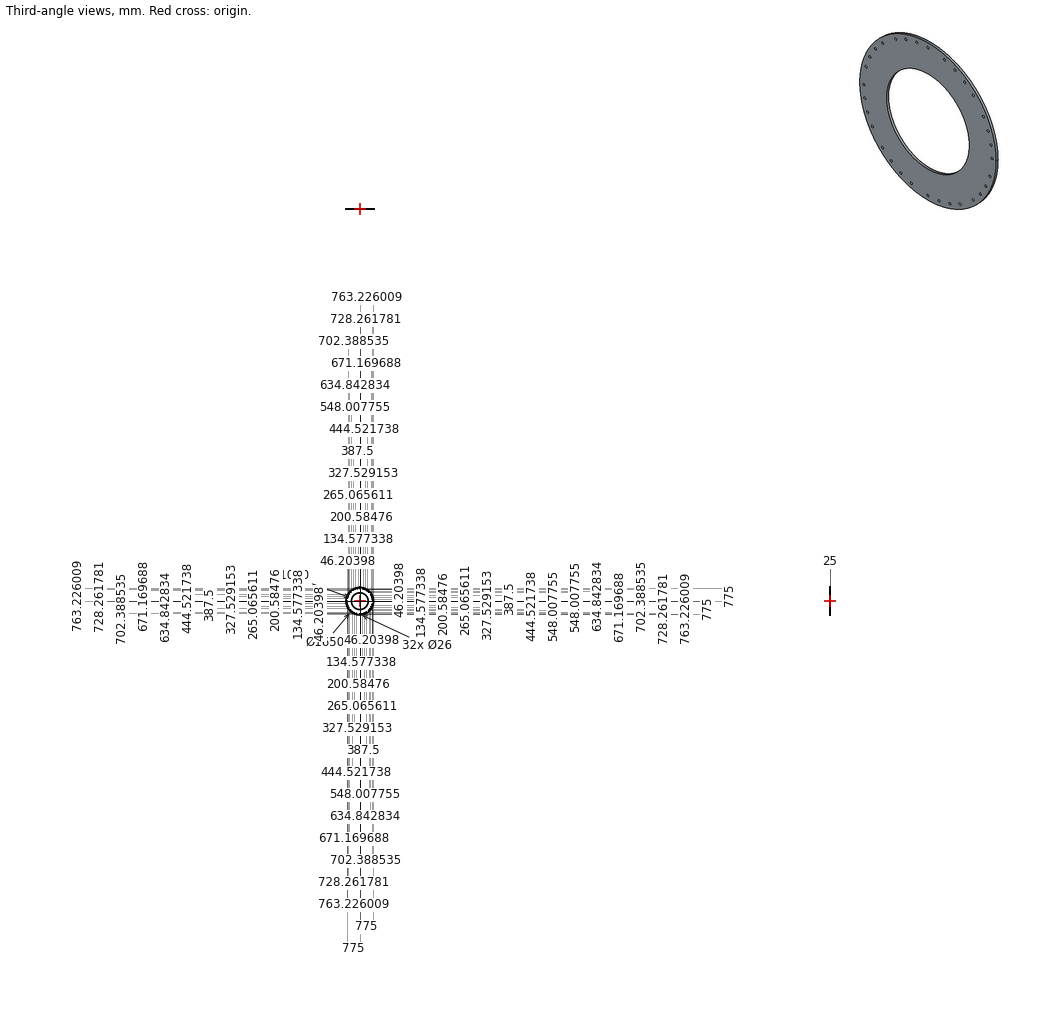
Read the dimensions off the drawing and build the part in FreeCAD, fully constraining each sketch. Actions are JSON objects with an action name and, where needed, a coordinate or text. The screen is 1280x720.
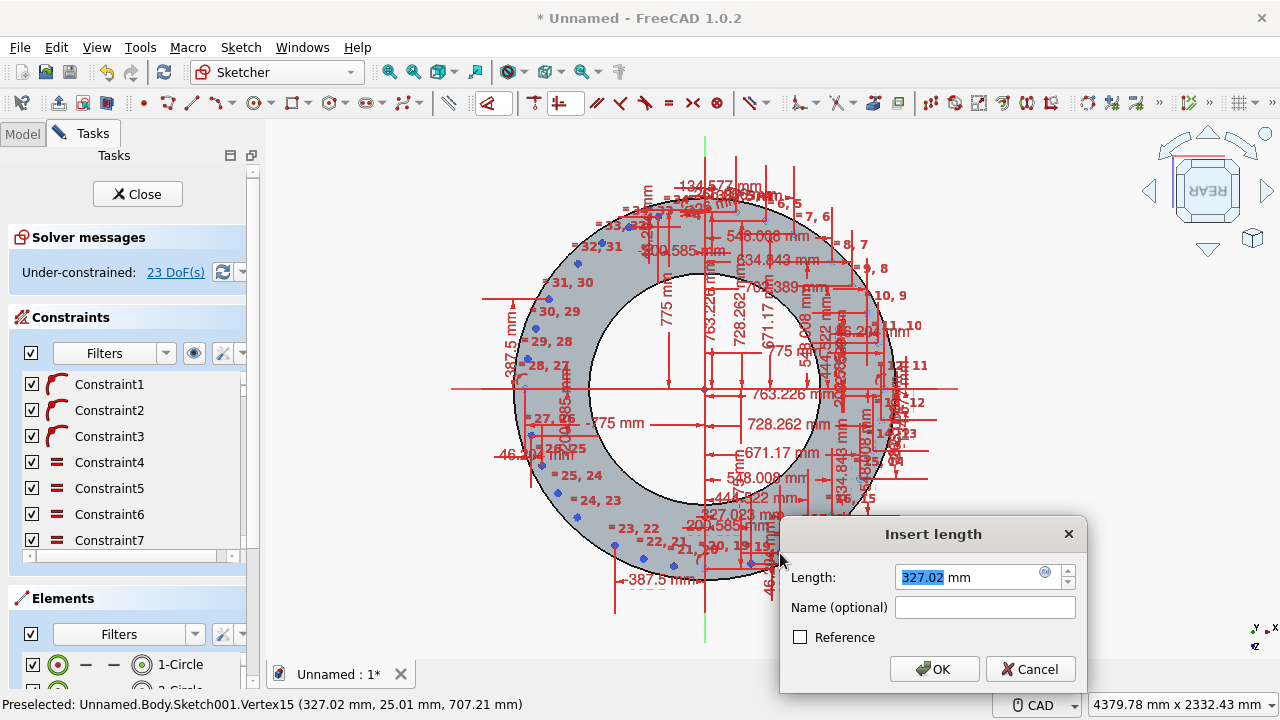
{"action": "type", "text": "327.529153"}
{"action": "key", "text": "Return"}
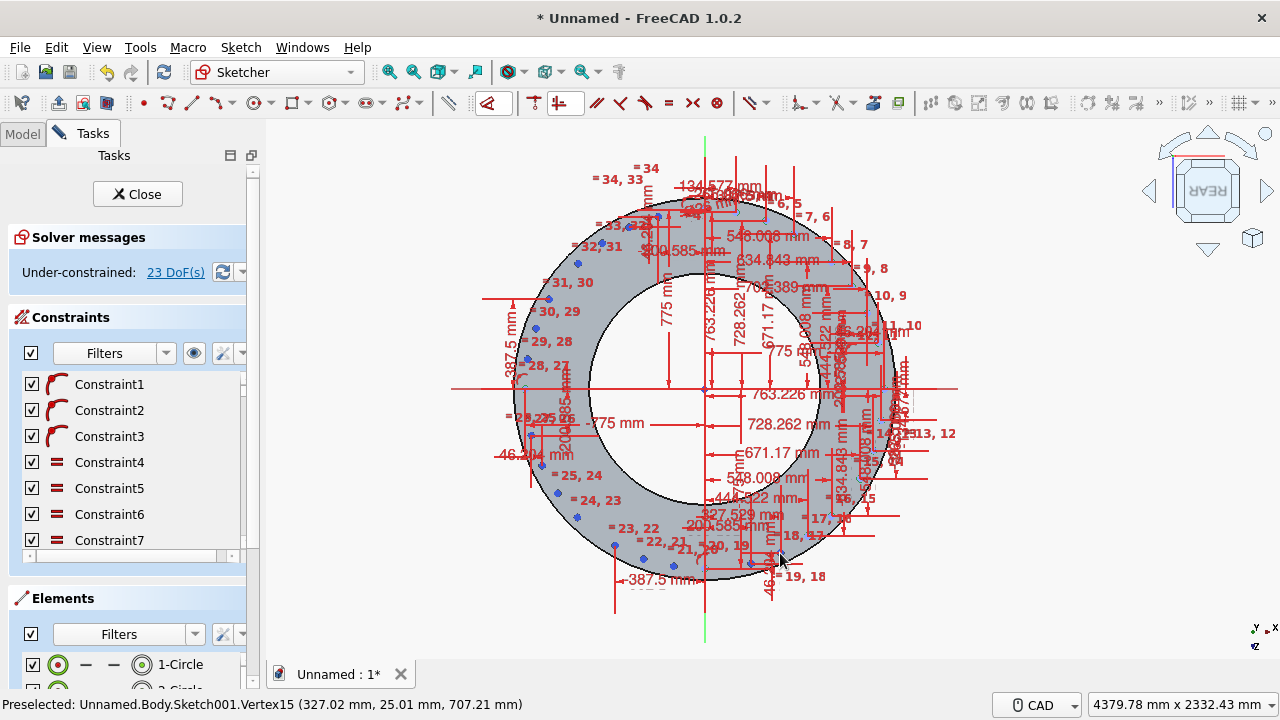
{"action": "left_click", "coordinate": [781, 553]}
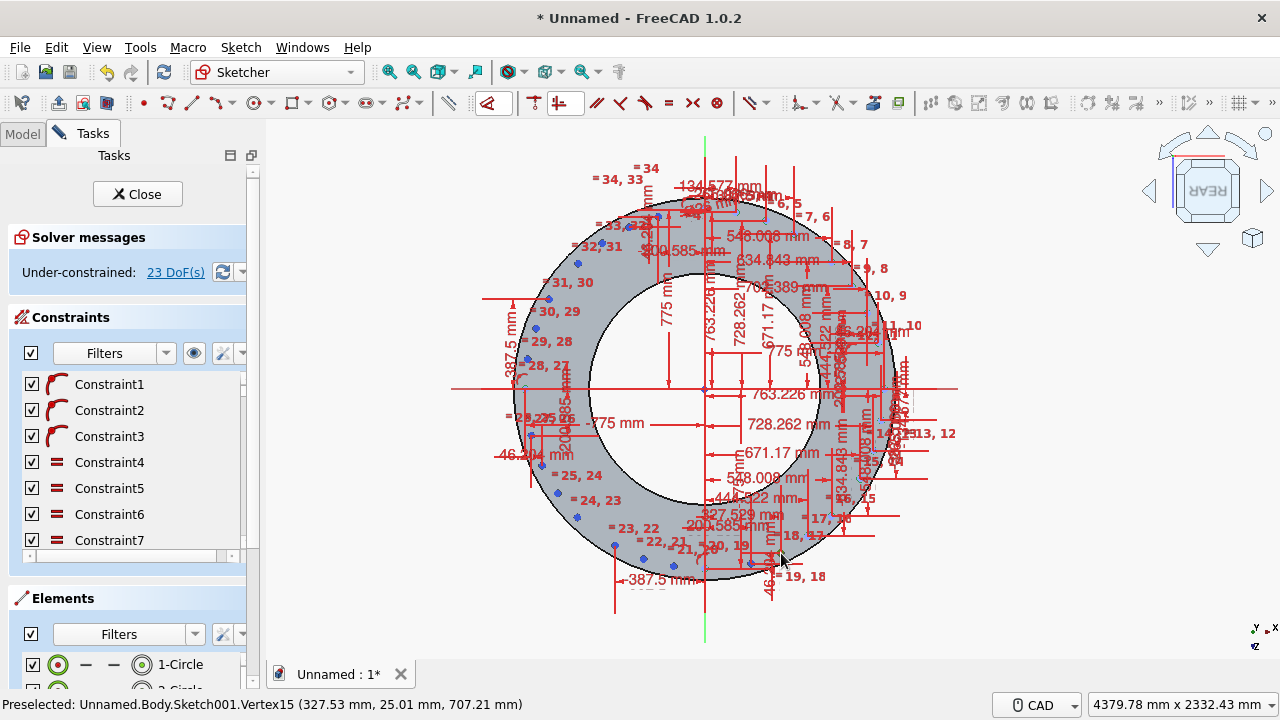
{"action": "key", "text": "i"}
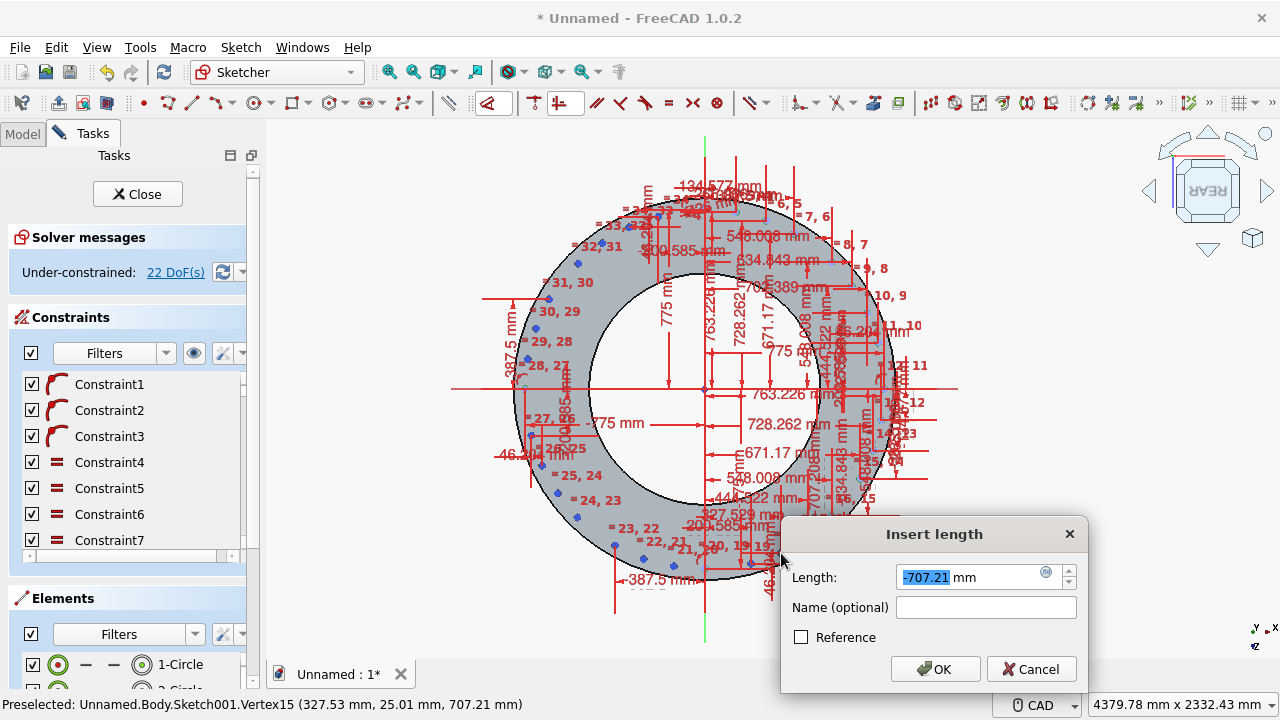
{"action": "type", "text": "-702.388535"}
{"action": "key", "text": "Return"}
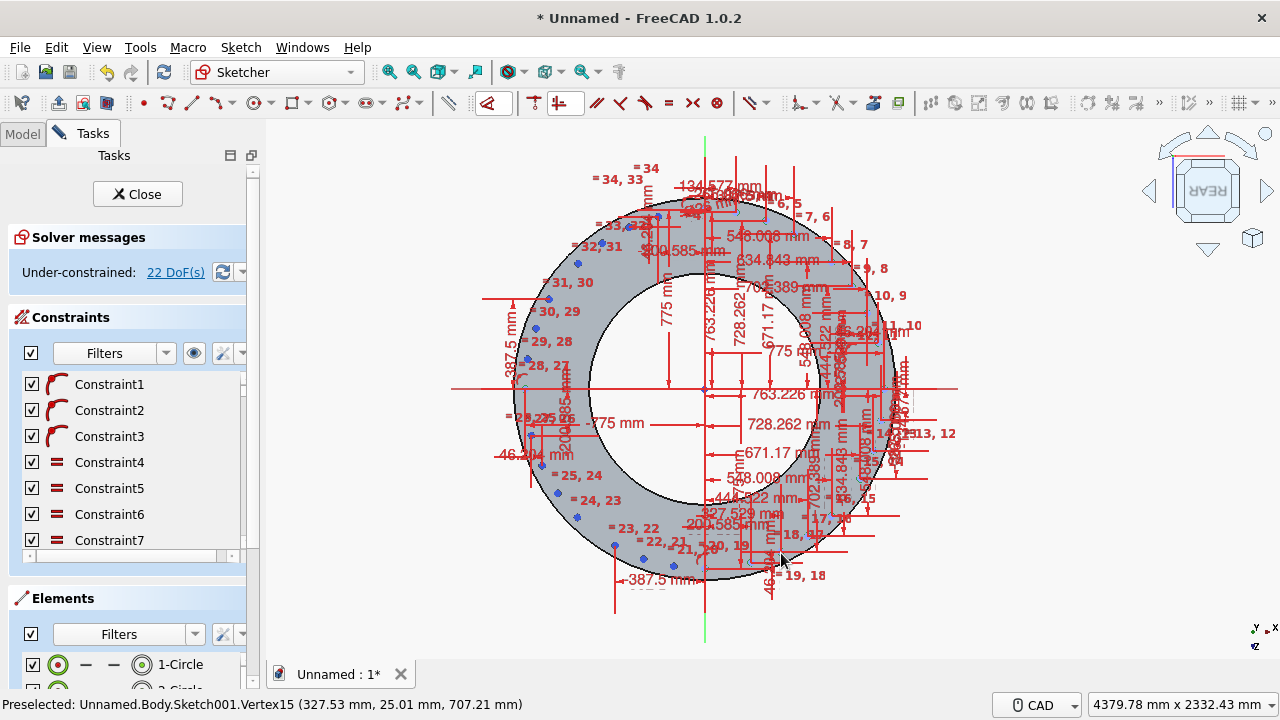
{"action": "scroll", "coordinate": [674, 566], "scroll_direction": "up", "scroll_amount": 2}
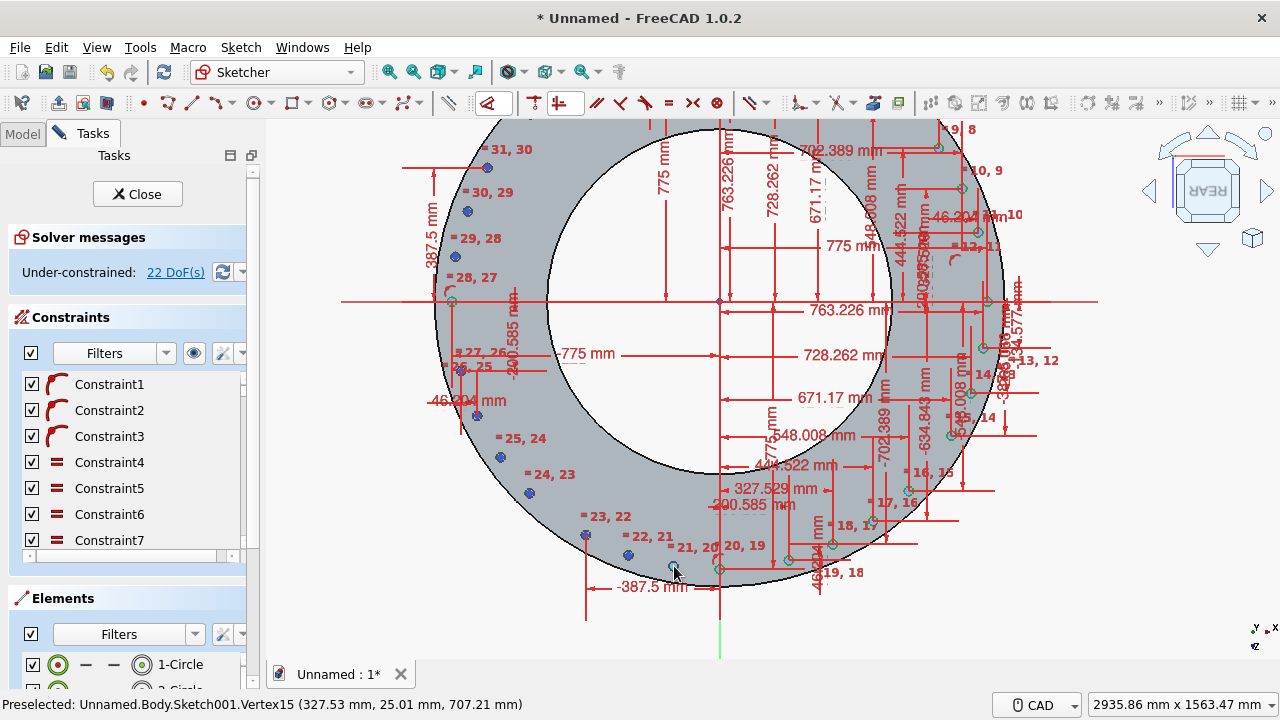
{"action": "left_click", "coordinate": [673, 566]}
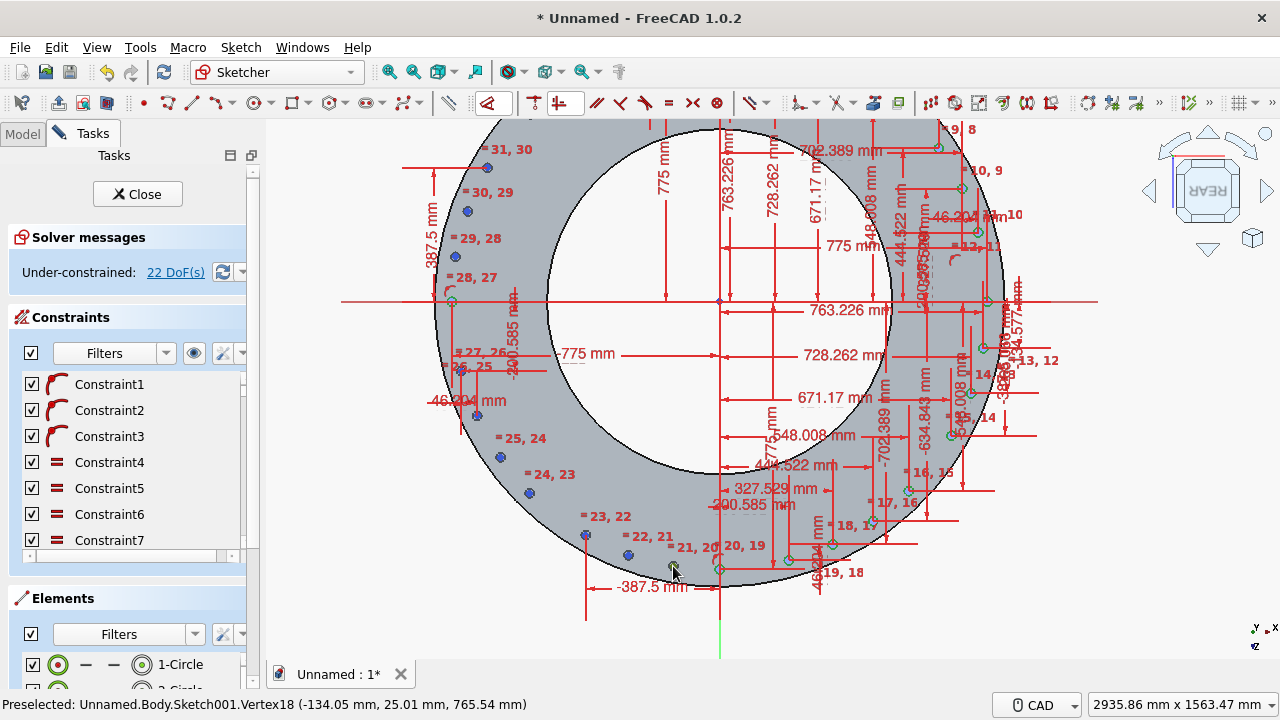
{"action": "key", "text": "l"}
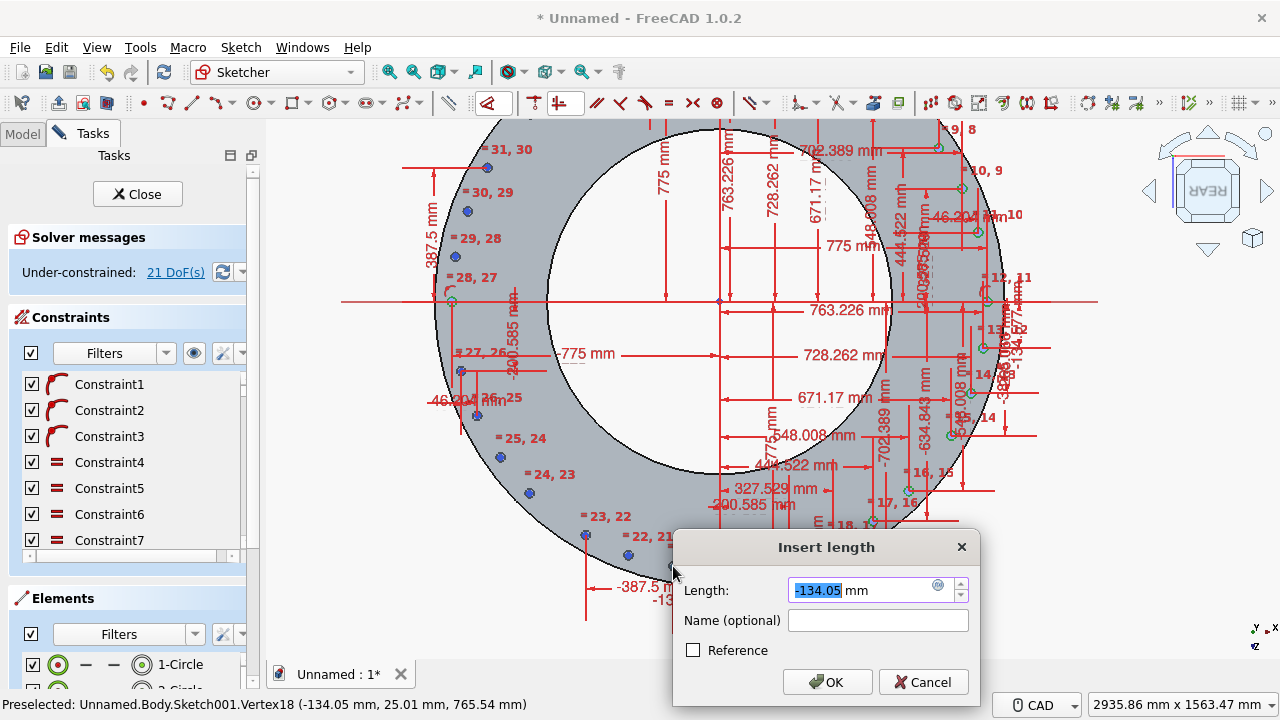
{"action": "type", "text": "-134.577338"}
{"action": "key", "text": "Return"}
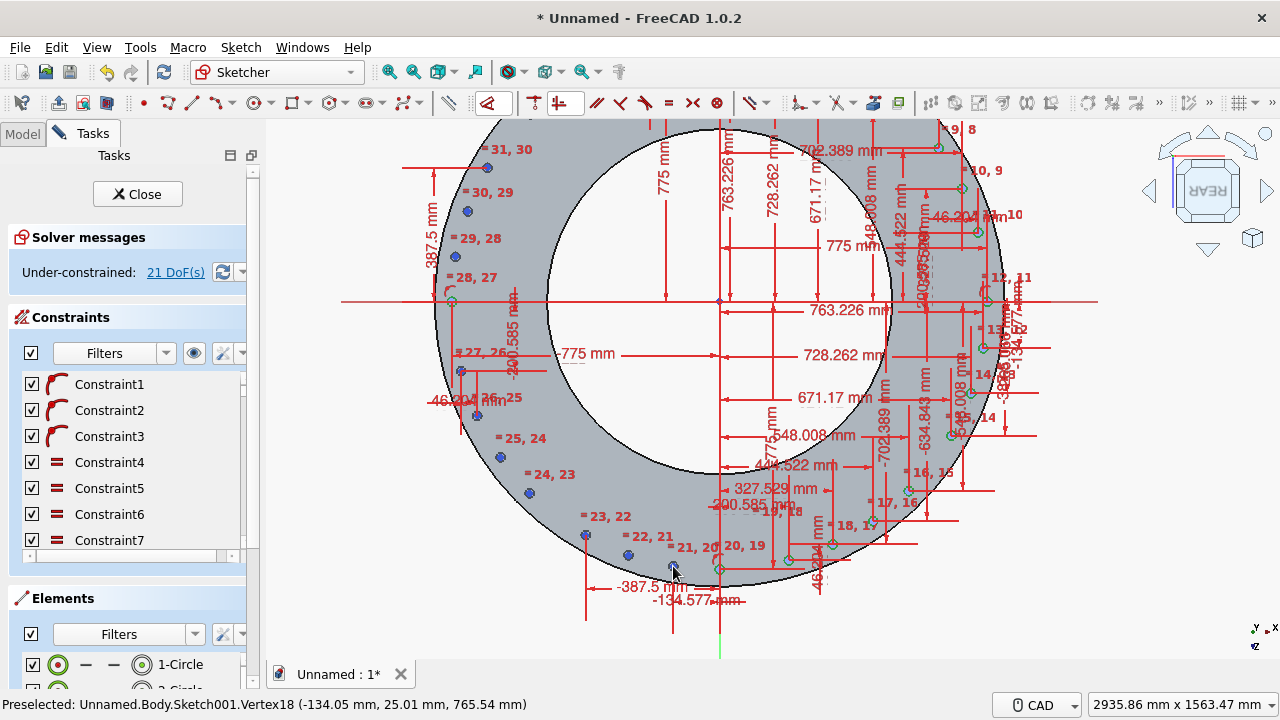
{"action": "left_click", "coordinate": [673, 566]}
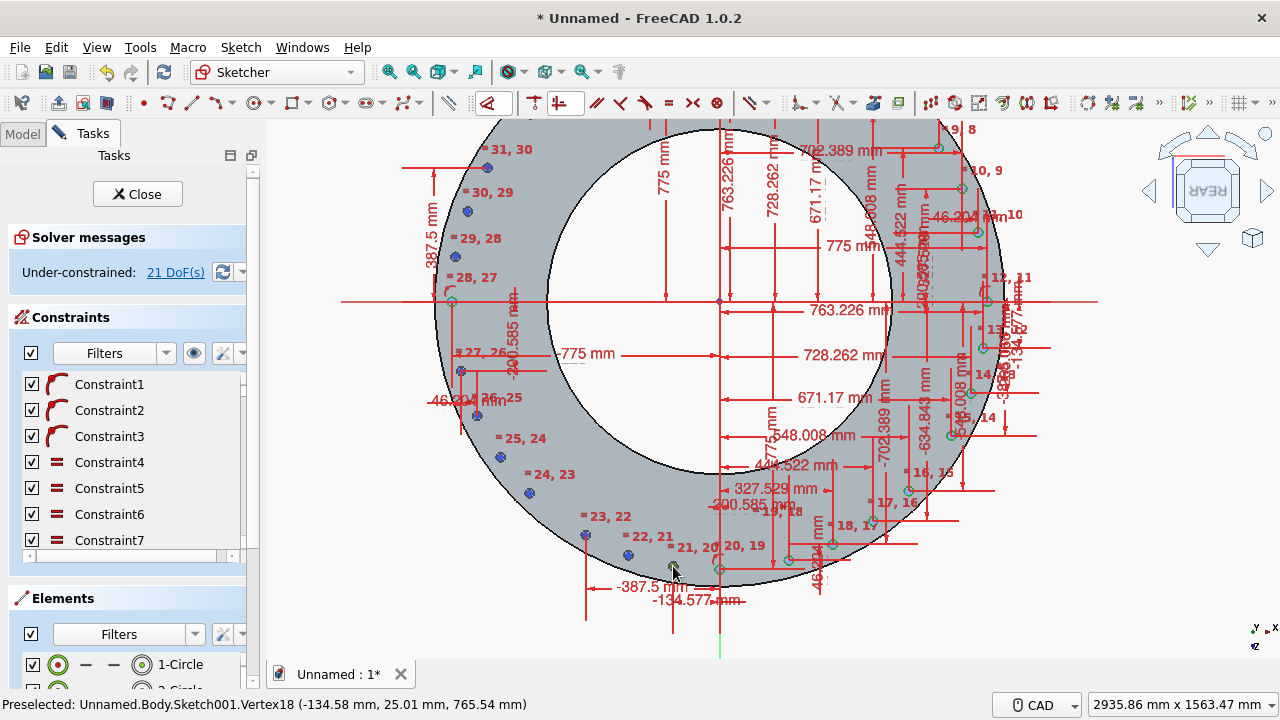
{"action": "key", "text": "i"}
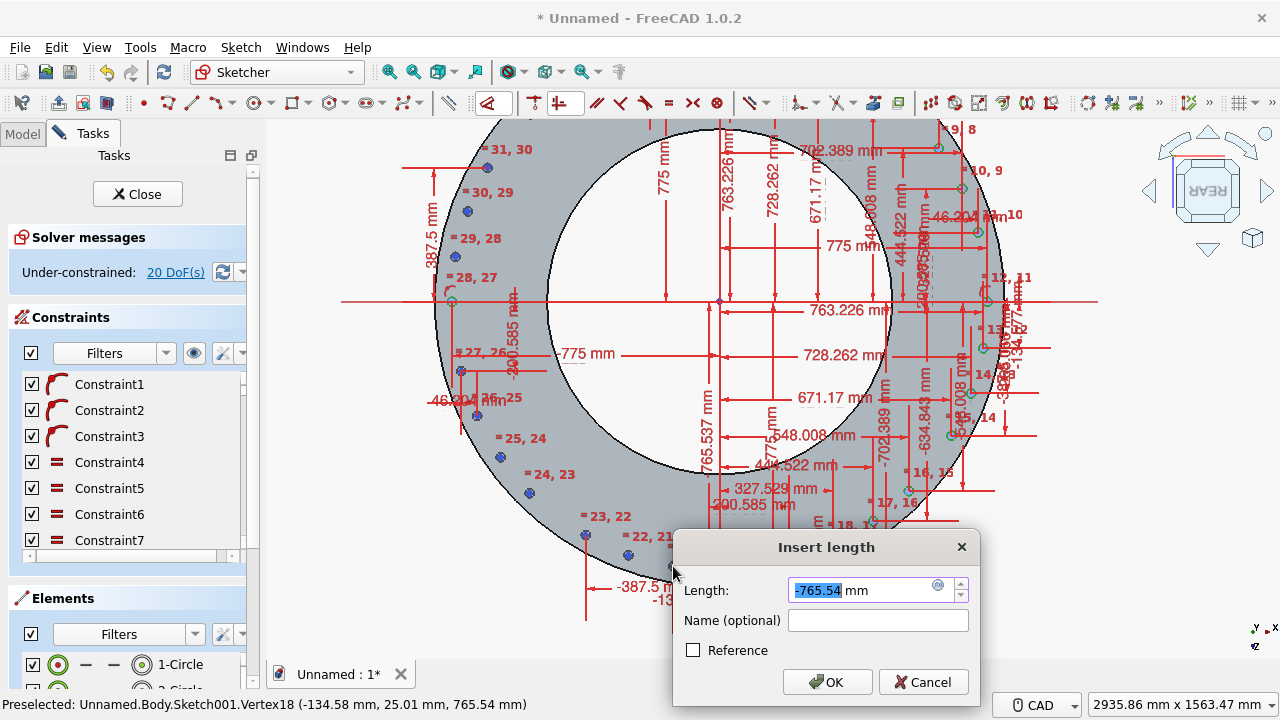
{"action": "type", "text": "-763.226009"}
{"action": "key", "text": "Return"}